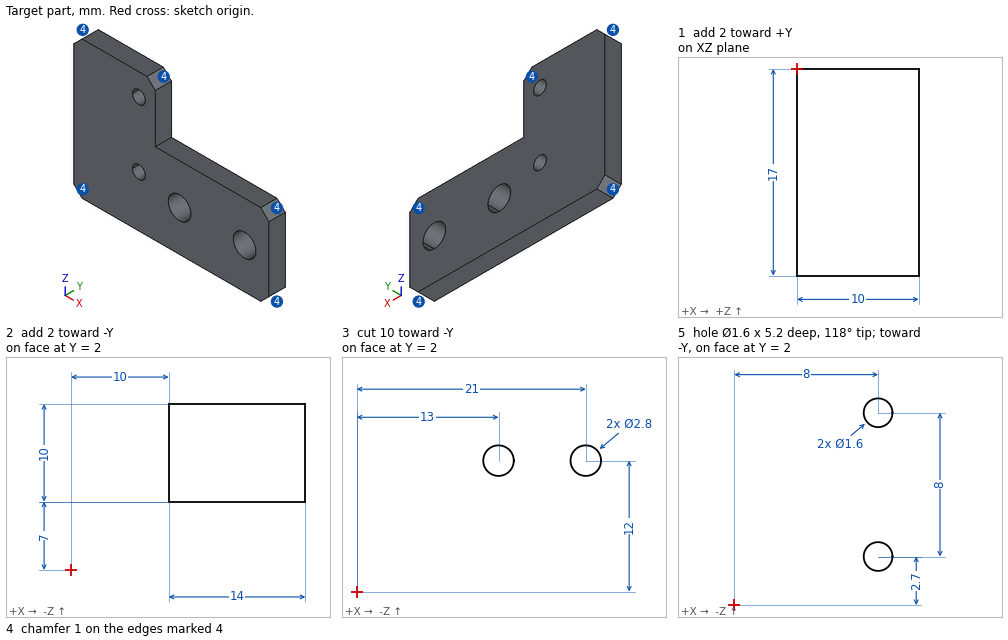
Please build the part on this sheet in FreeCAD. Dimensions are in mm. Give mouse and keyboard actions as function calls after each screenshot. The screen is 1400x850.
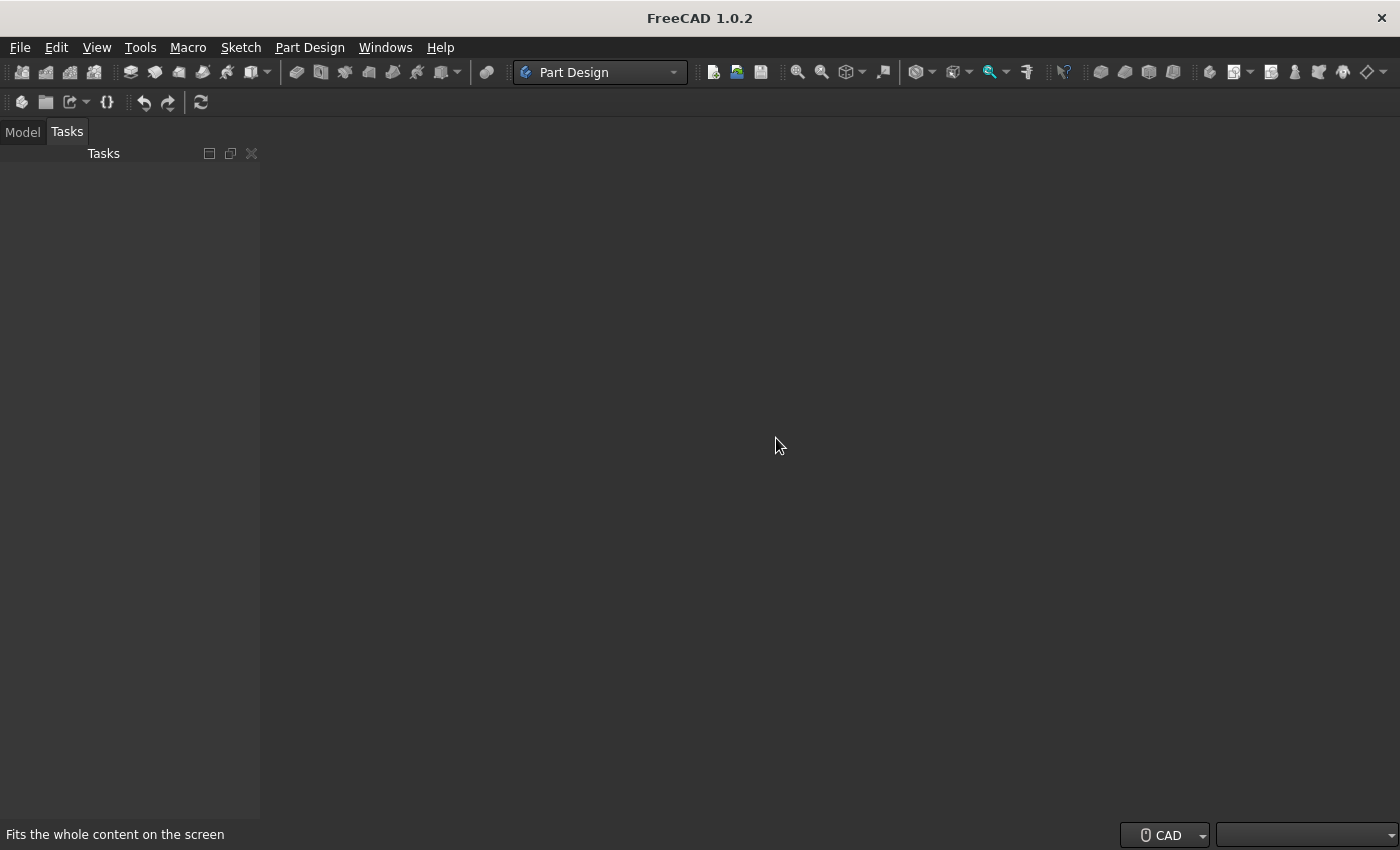
click(714, 72)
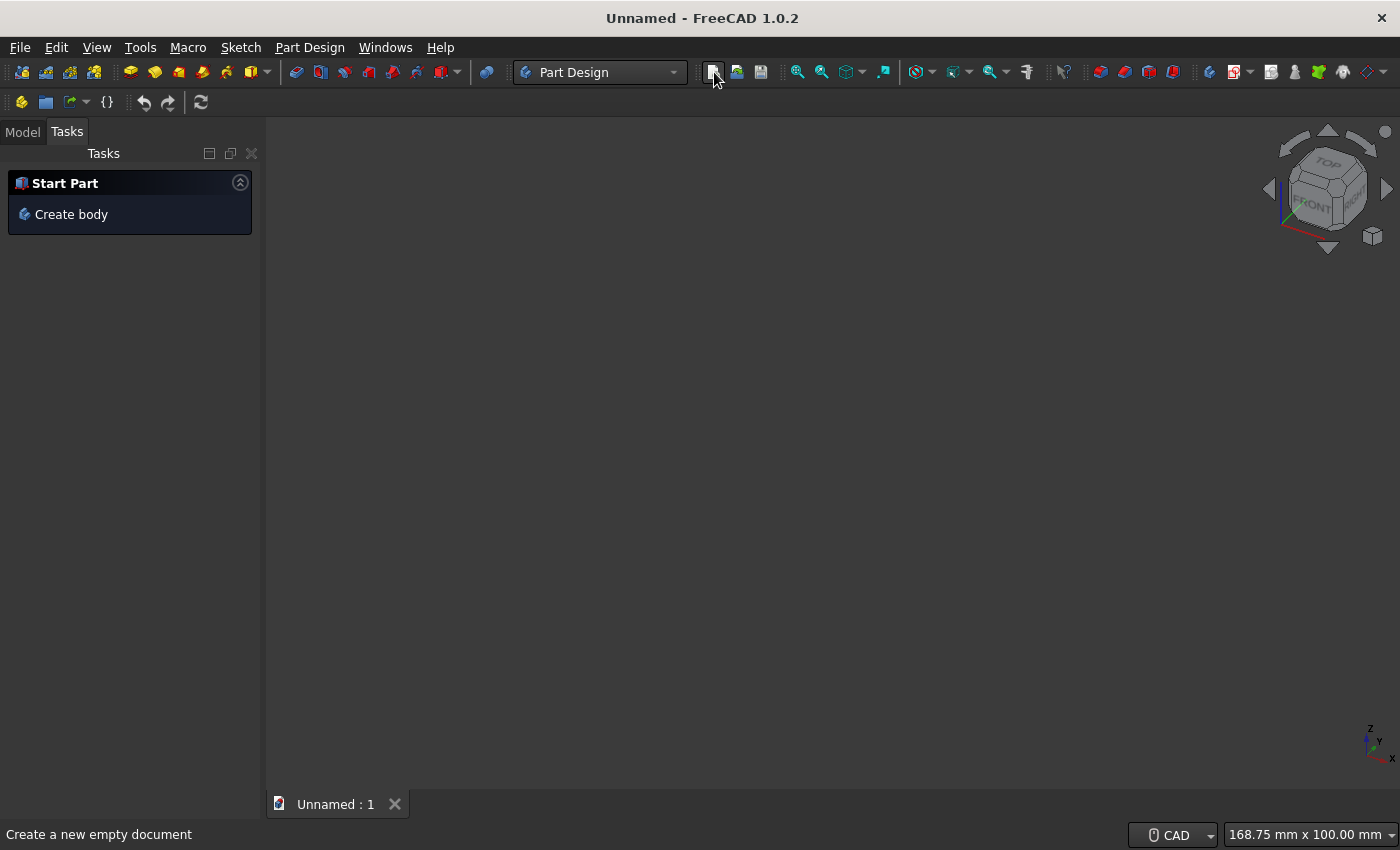
click(1234, 72)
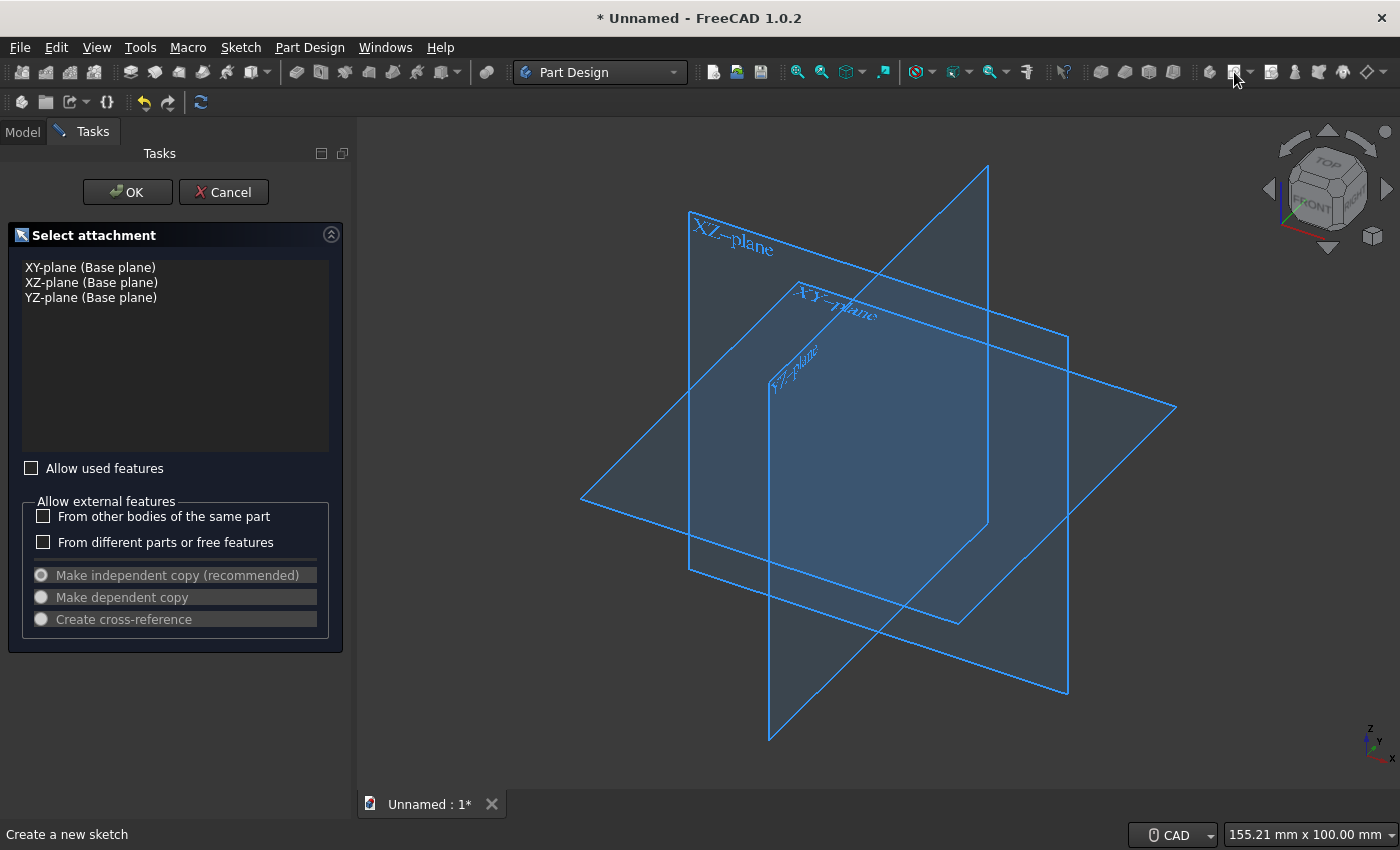
click(82, 282)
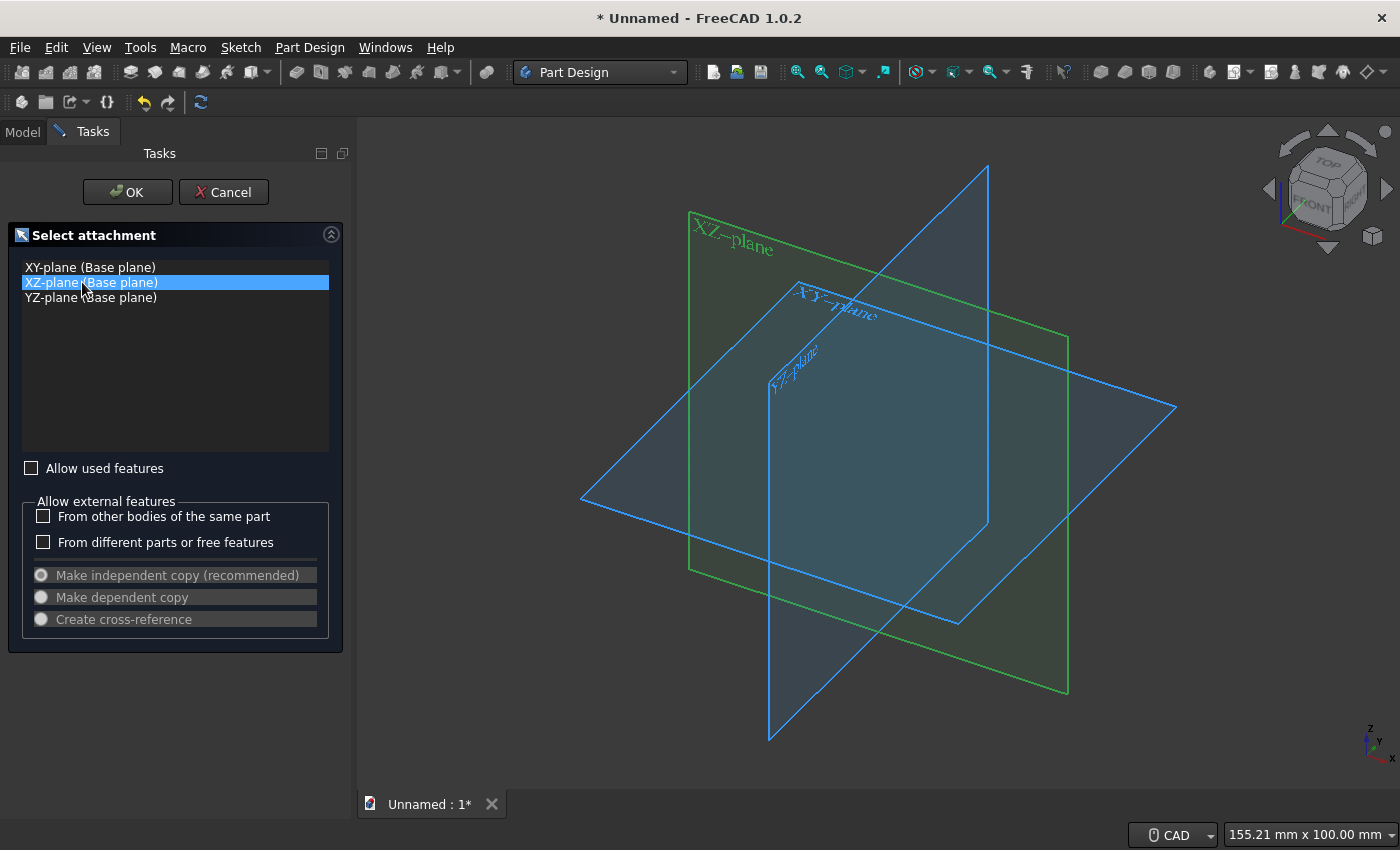
click(128, 192)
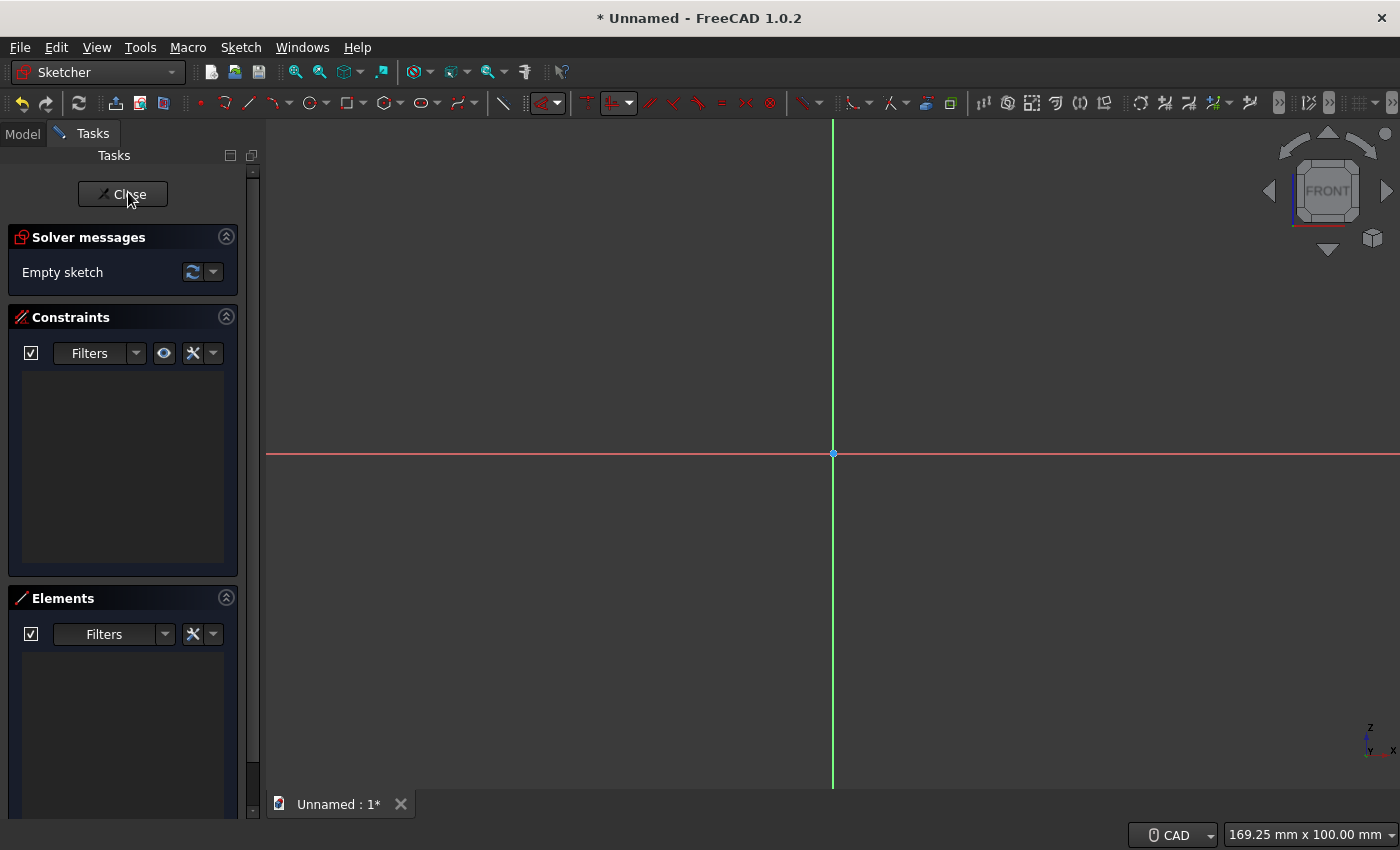
scroll(900, 530, up, 7)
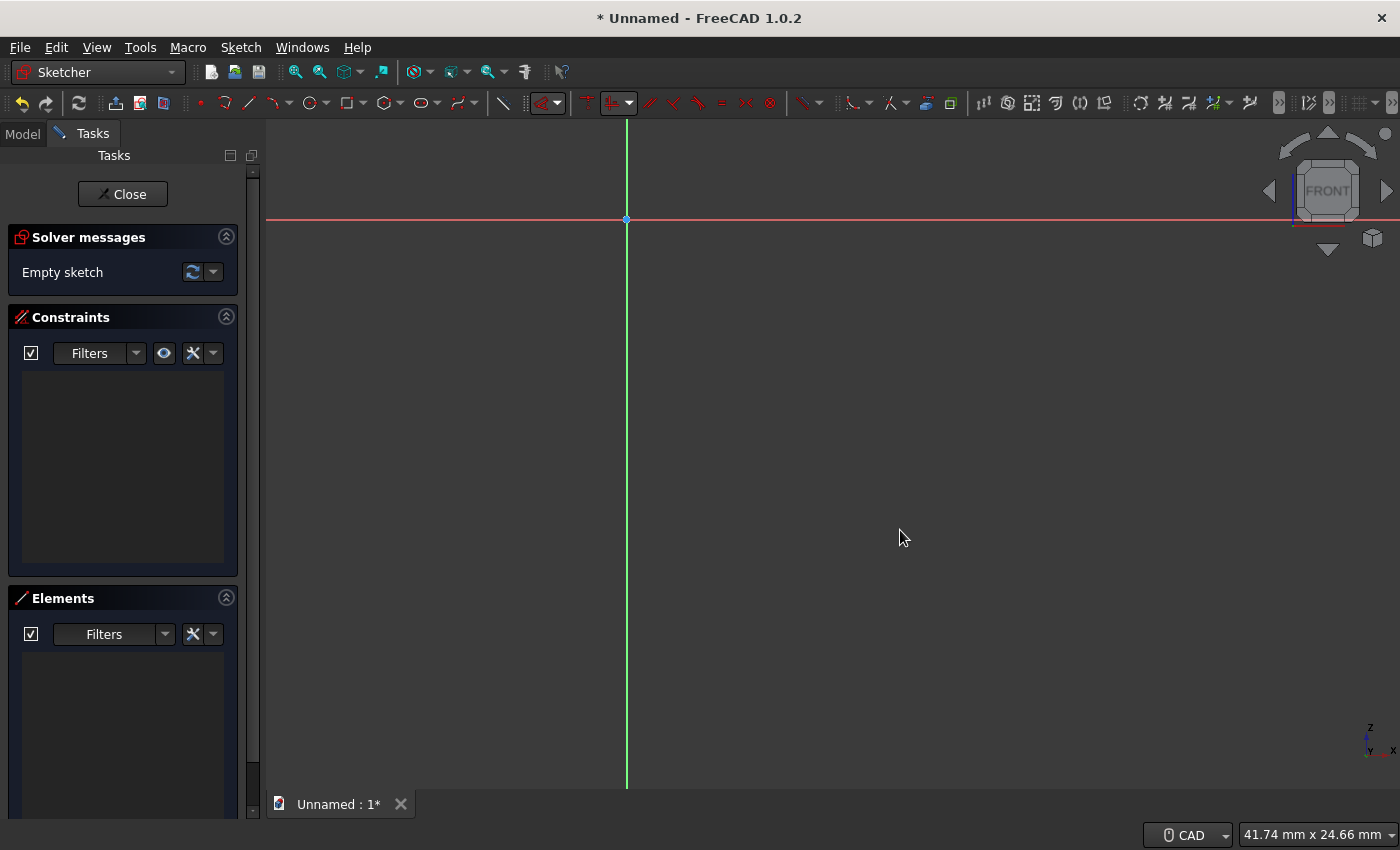
click(348, 104)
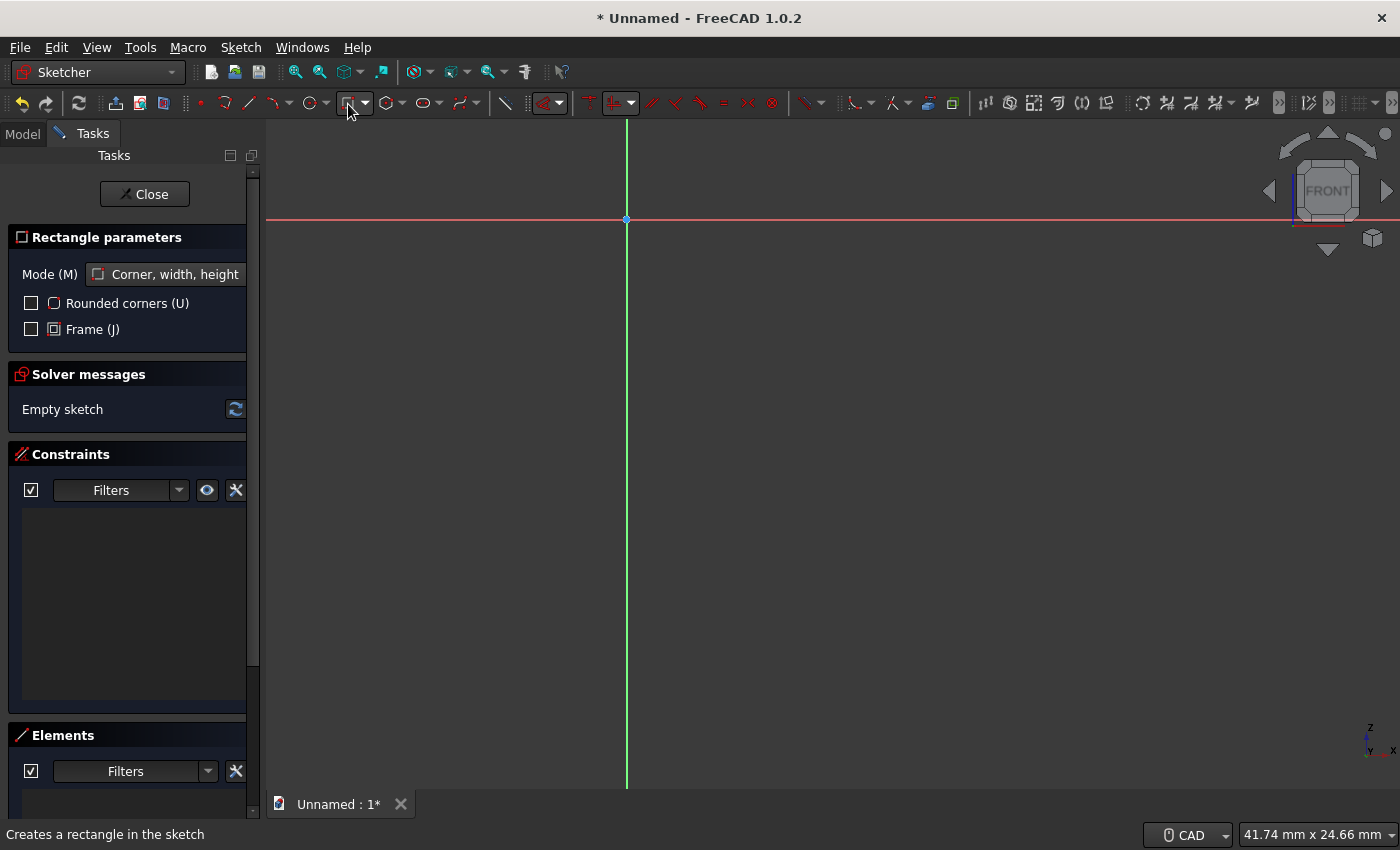
click(627, 220)
click(898, 682)
key(Escape)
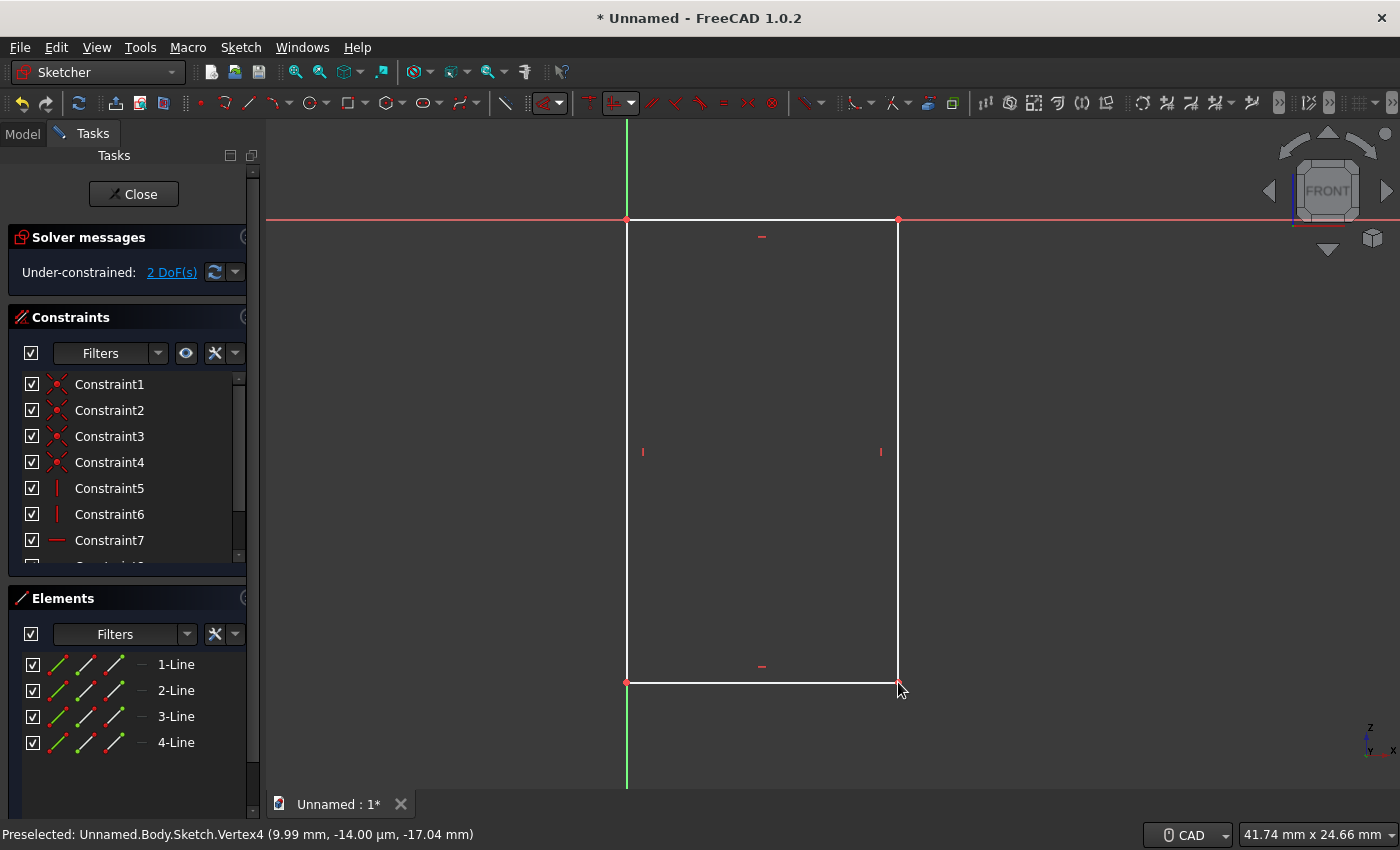
click(627, 359)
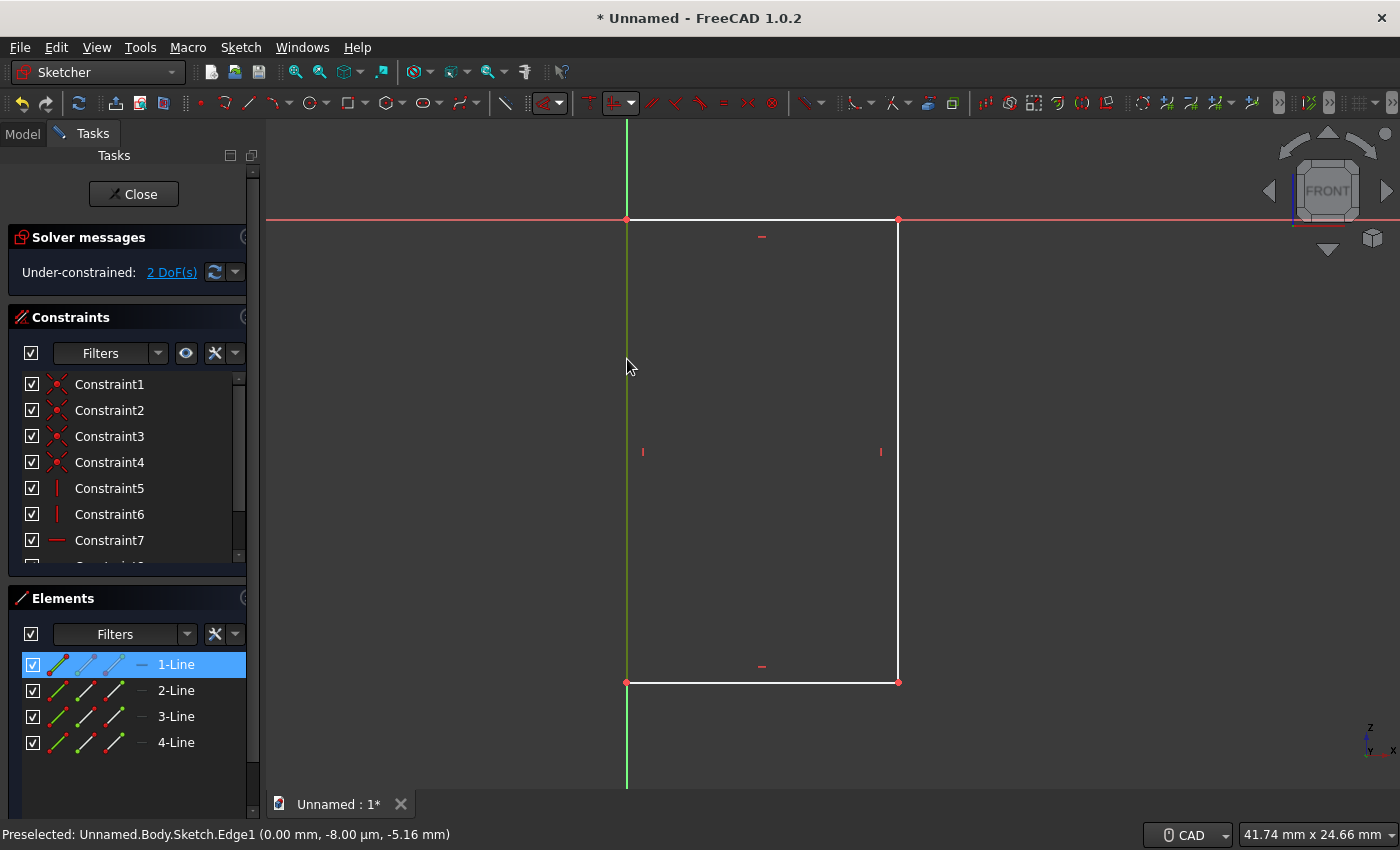
click(562, 104)